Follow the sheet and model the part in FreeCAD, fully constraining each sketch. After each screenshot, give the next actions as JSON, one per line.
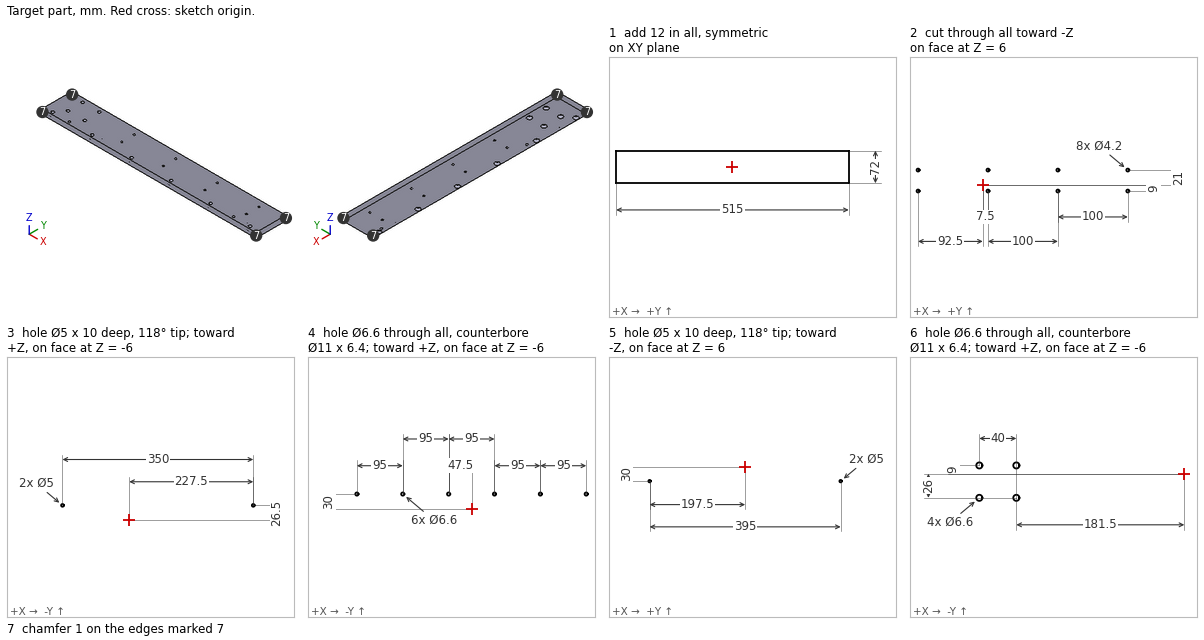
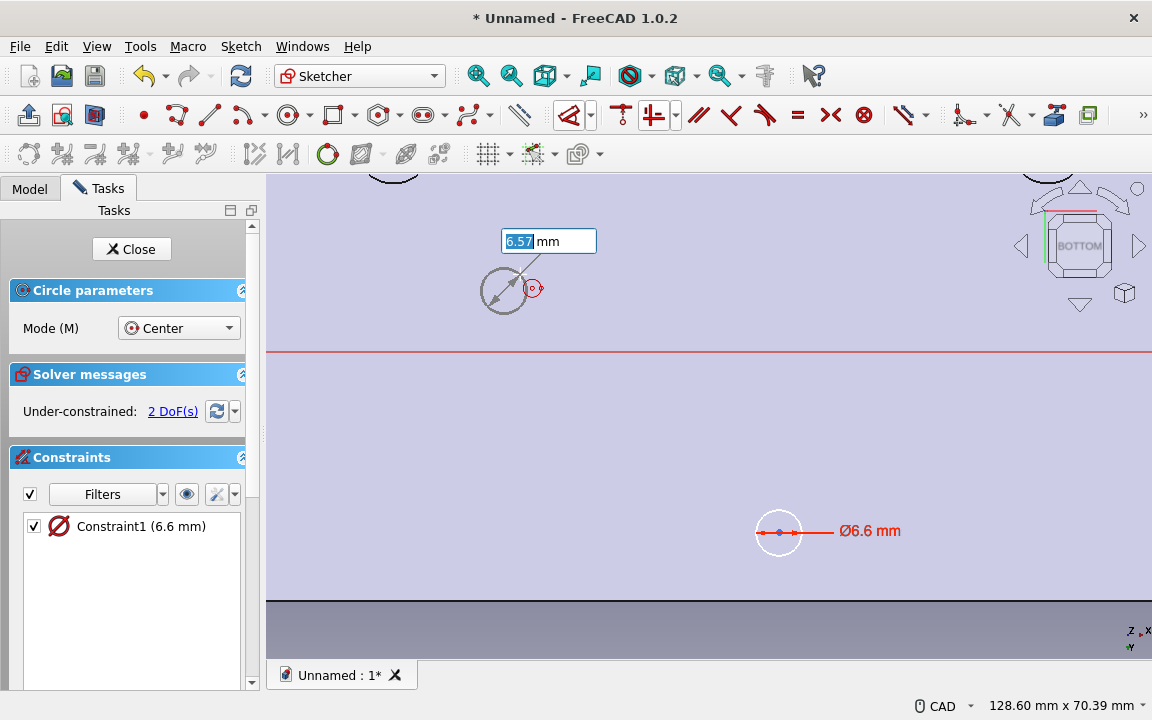
{"action": "type", "text": "6.6"}
{"action": "key", "text": "Return"}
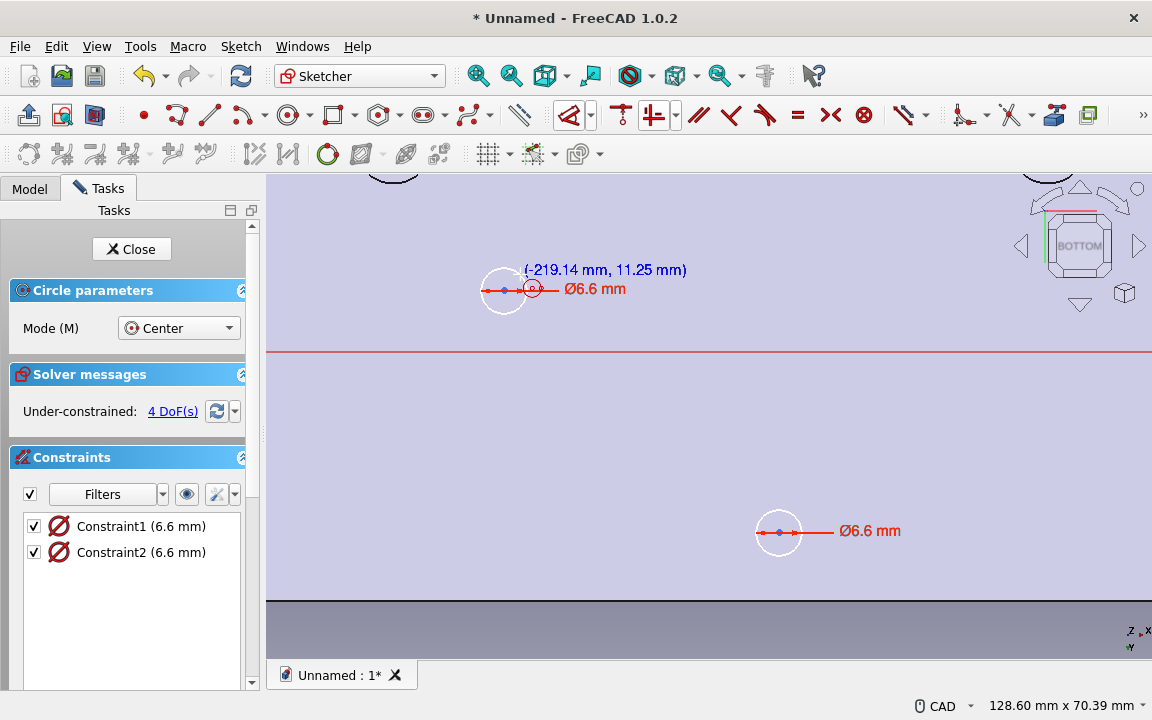
{"action": "left_click", "coordinate": [779, 290]}
{"action": "mouse_move", "coordinate": [795, 274]}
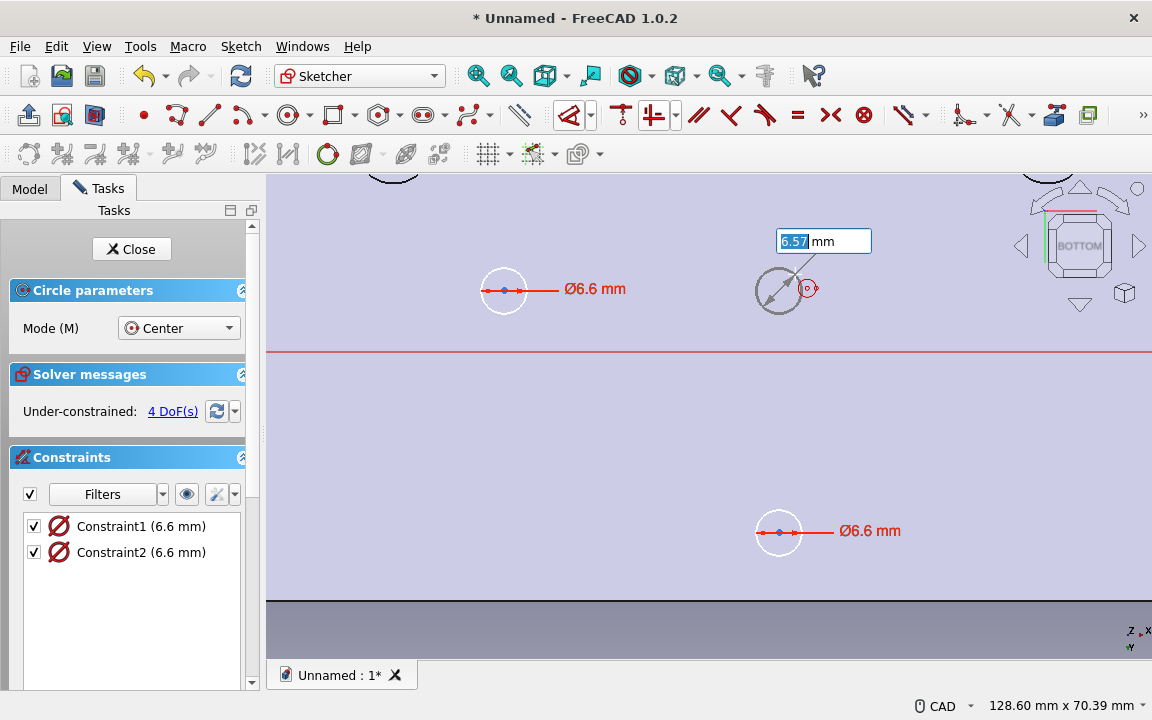
{"action": "type", "text": "6.6"}
{"action": "key", "text": "Return"}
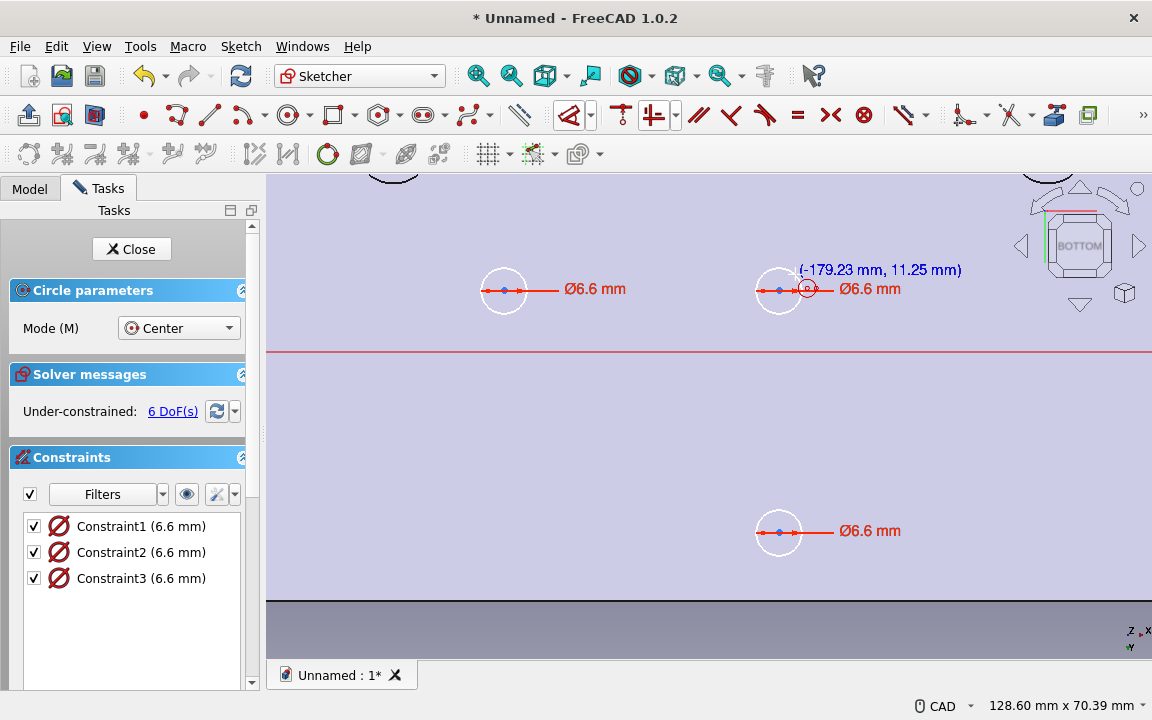
{"action": "left_click", "coordinate": [504, 532]}
{"action": "mouse_move", "coordinate": [520, 516]}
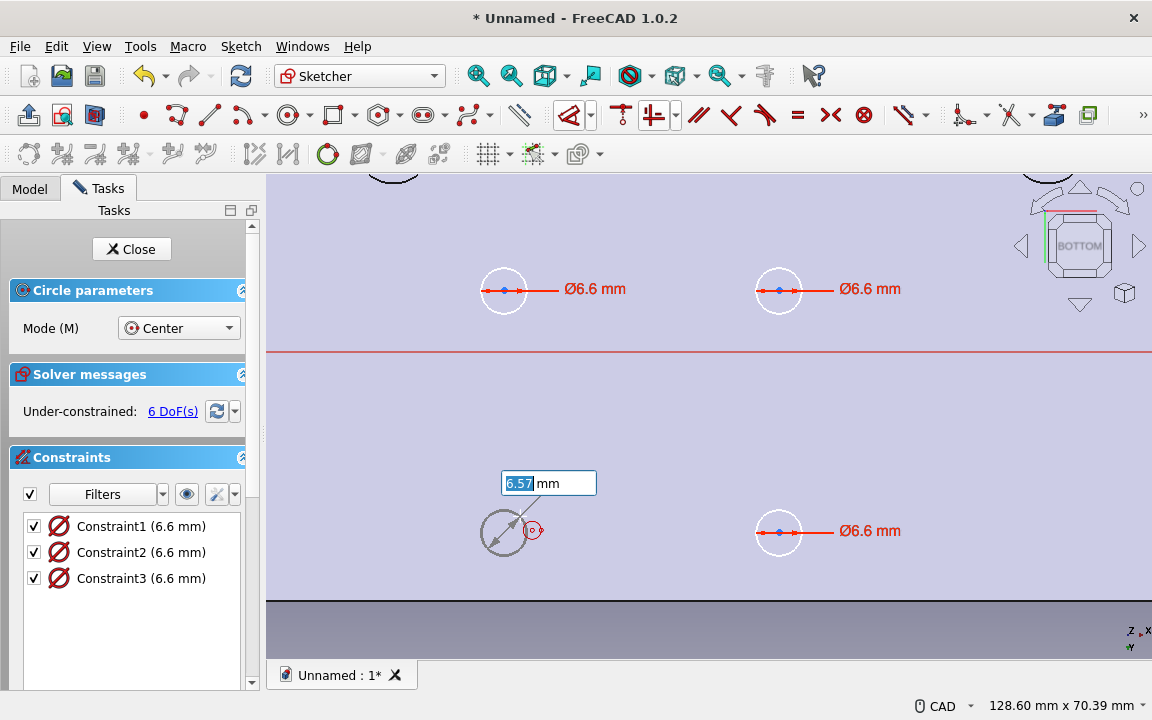
{"action": "type", "text": "6.6"}
{"action": "key", "text": "Return"}
{"action": "key", "text": "Escape"}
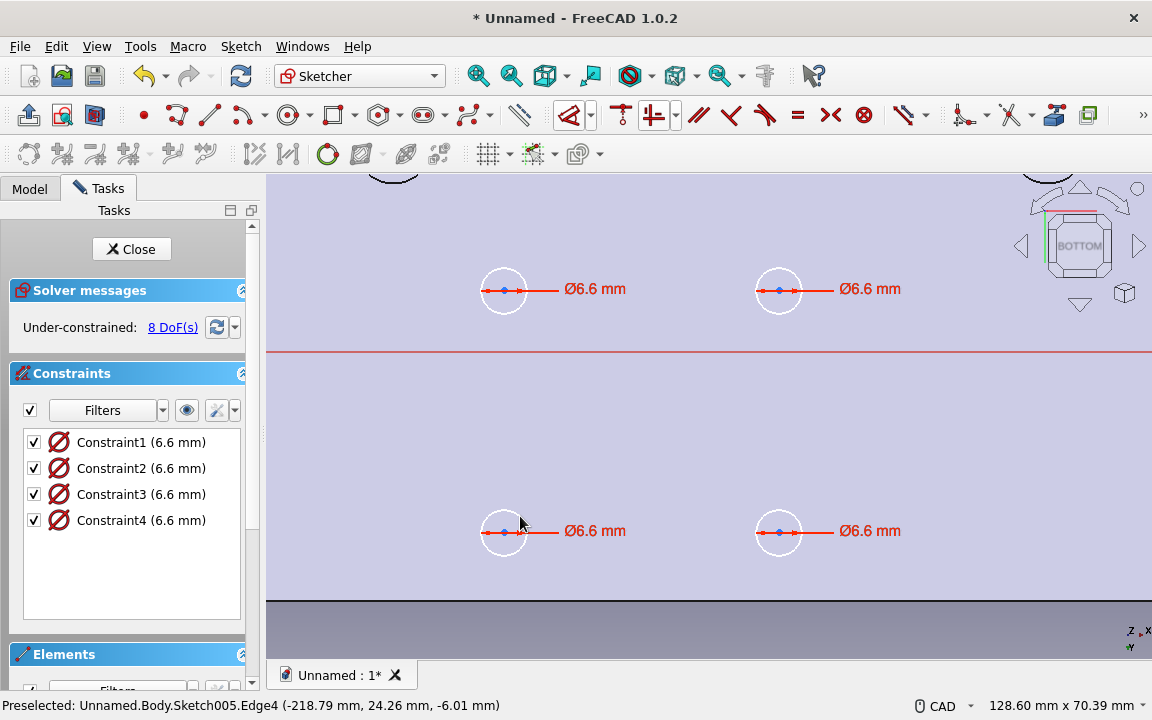
{"action": "left_click", "coordinate": [779, 533]}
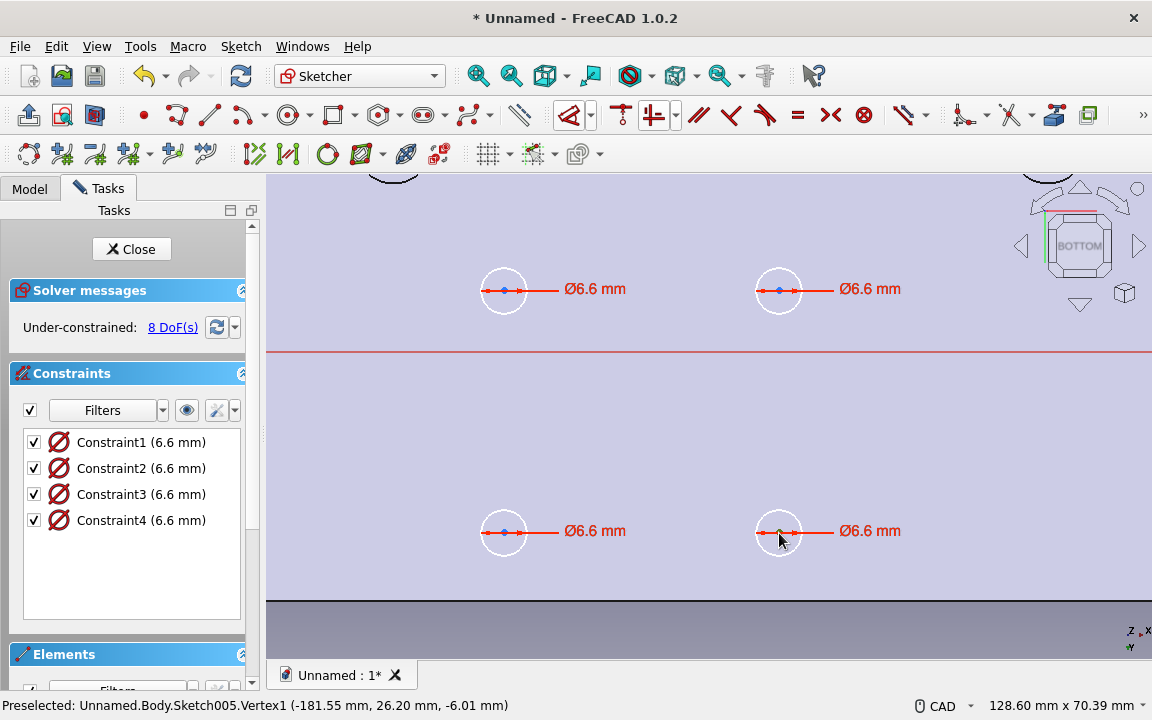
{"action": "left_click", "coordinate": [779, 291]}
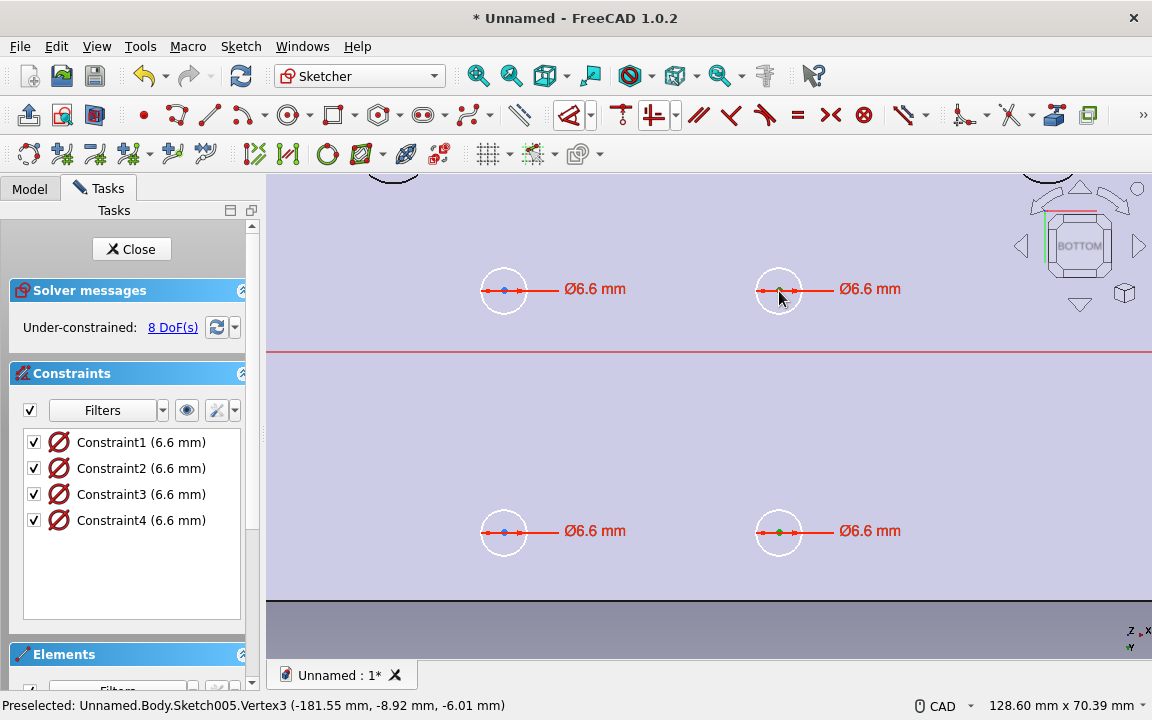
{"action": "left_click", "coordinate": [676, 116]}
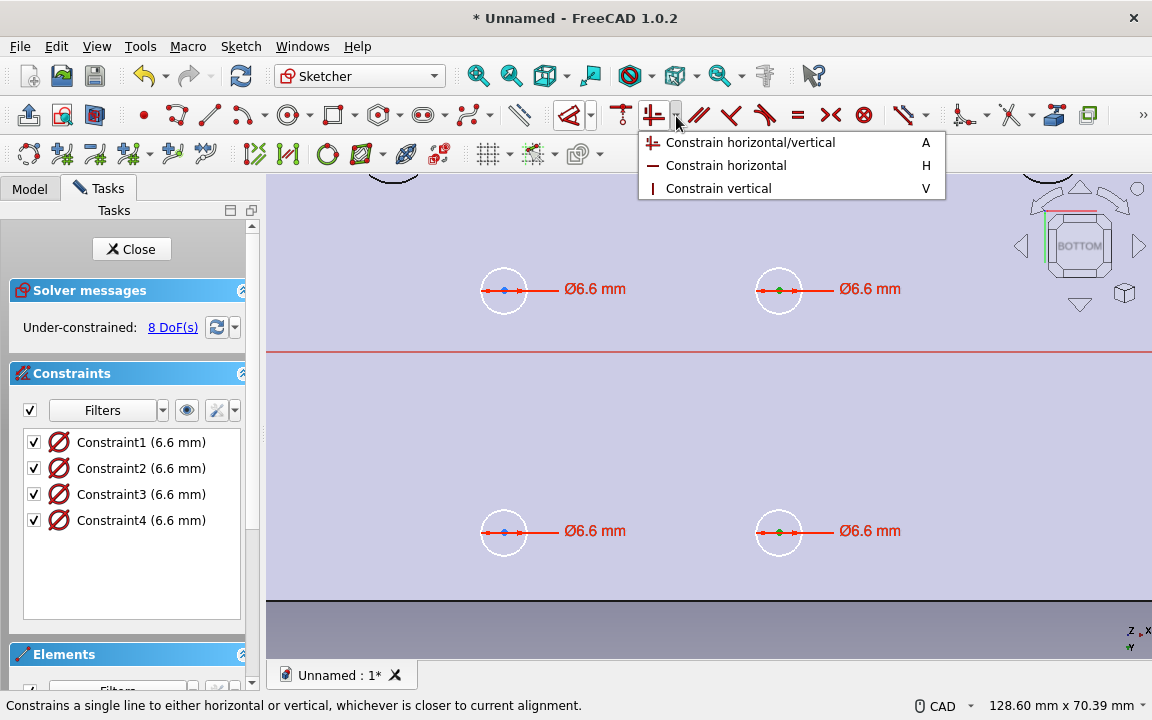
{"action": "left_click", "coordinate": [792, 188]}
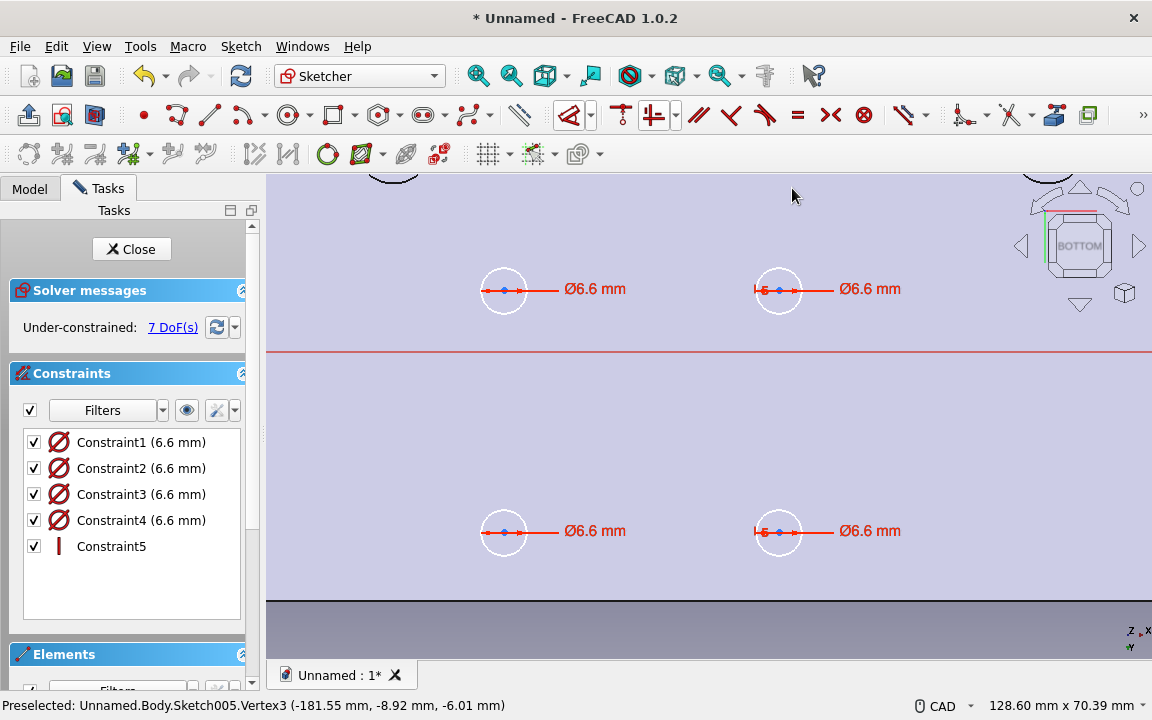
{"action": "left_click", "coordinate": [504, 291]}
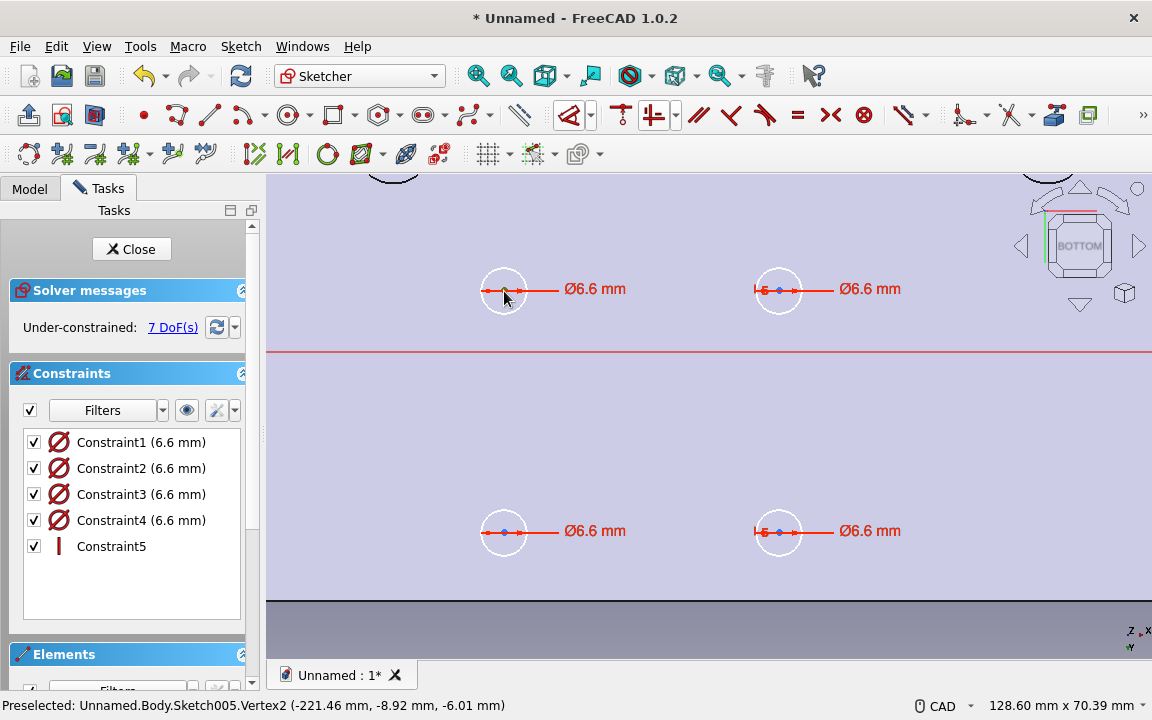
{"action": "left_click", "coordinate": [779, 291]}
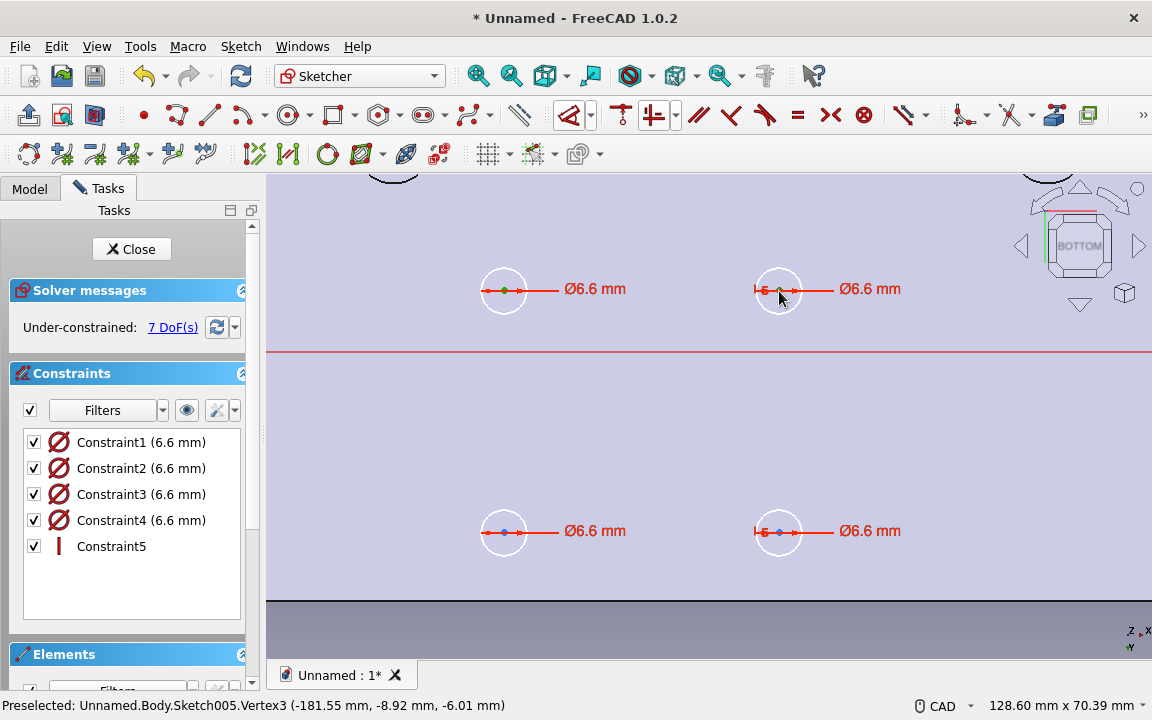
{"action": "left_click", "coordinate": [676, 116]}